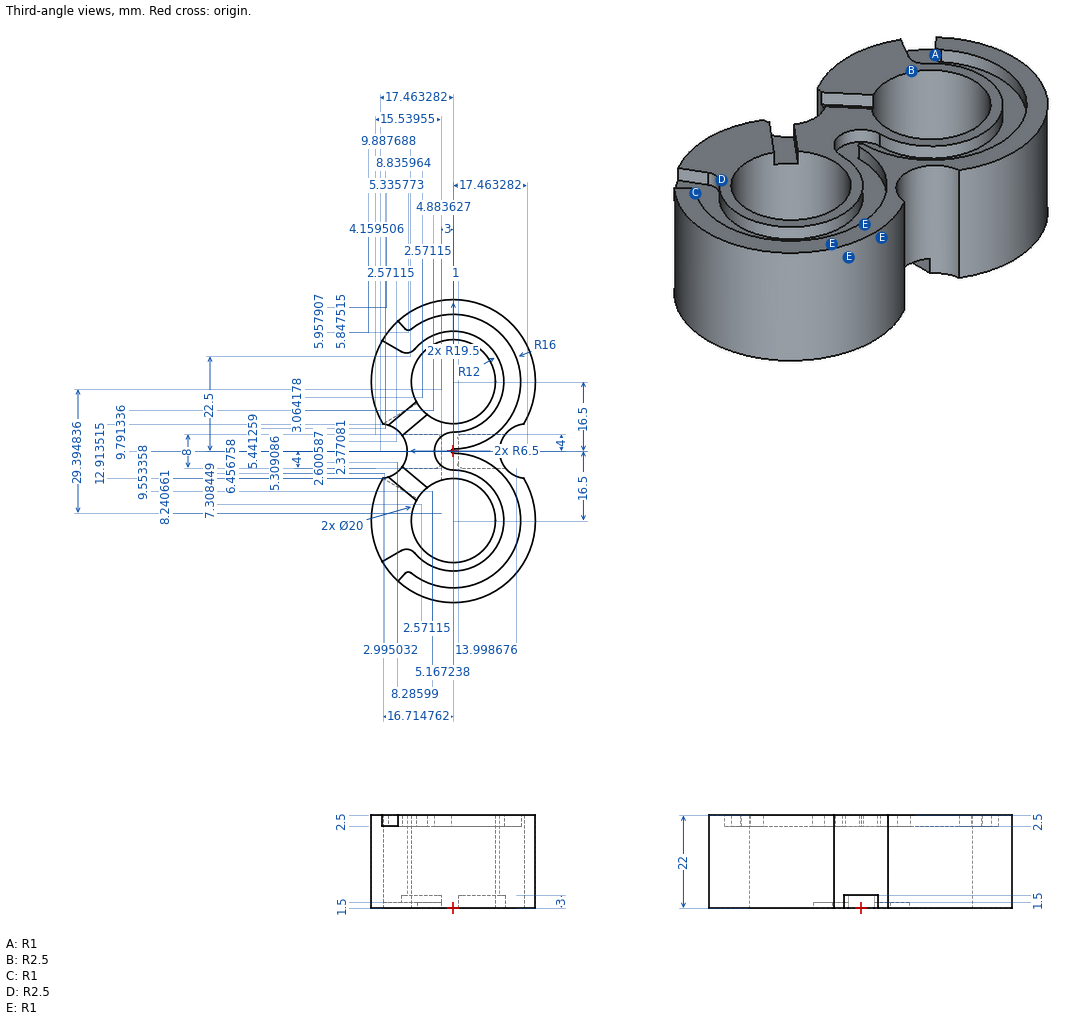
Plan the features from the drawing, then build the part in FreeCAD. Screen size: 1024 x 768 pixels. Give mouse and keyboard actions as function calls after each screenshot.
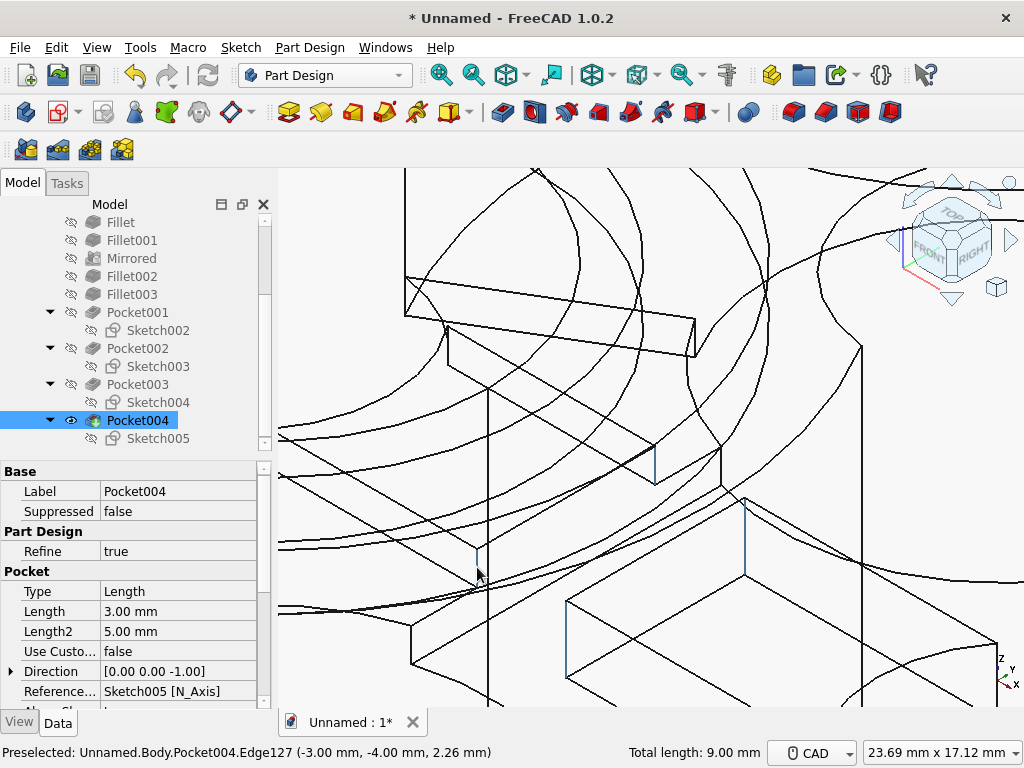
key(v)
key(1)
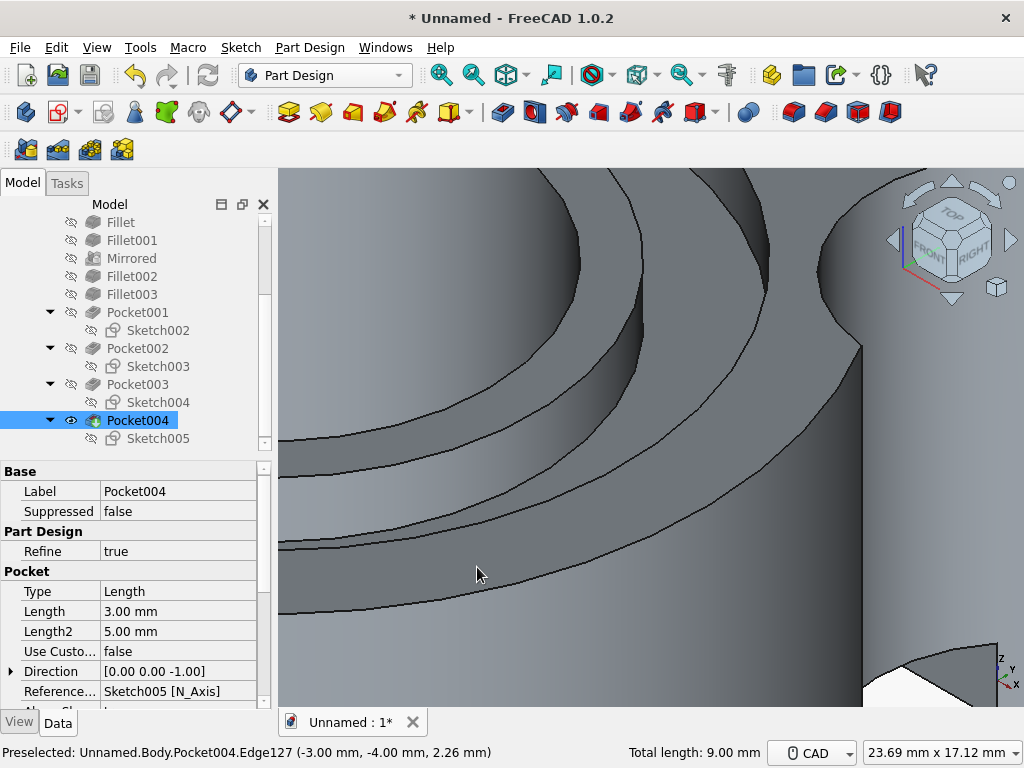
click(794, 112)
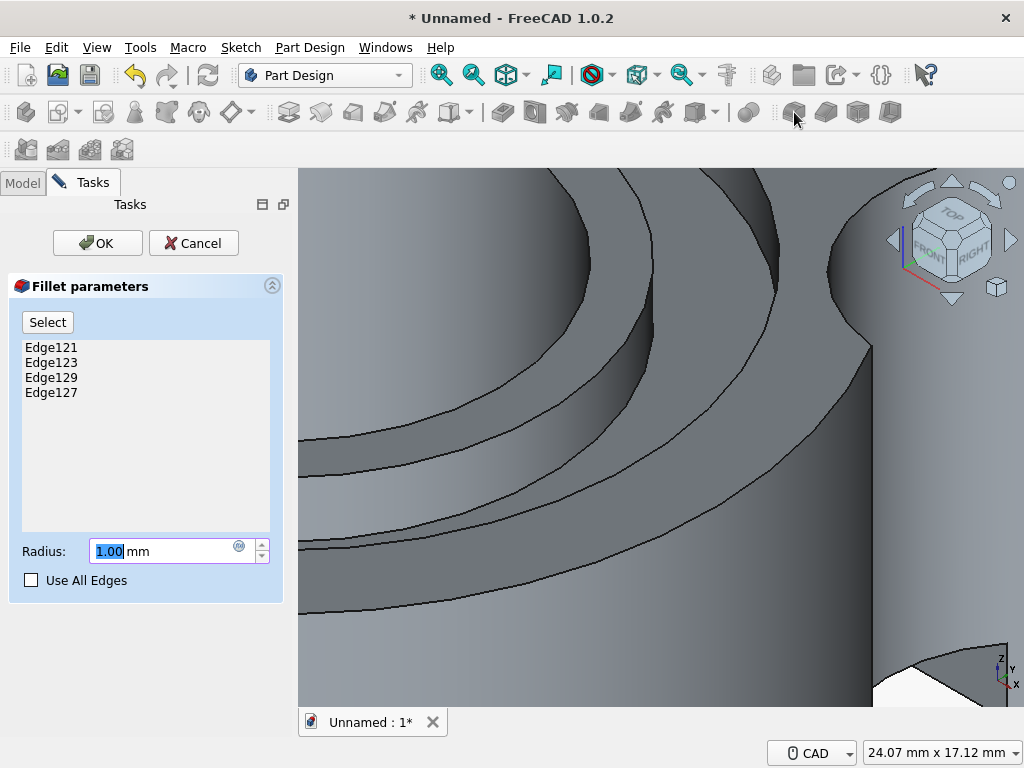
text(1)
key(Tab)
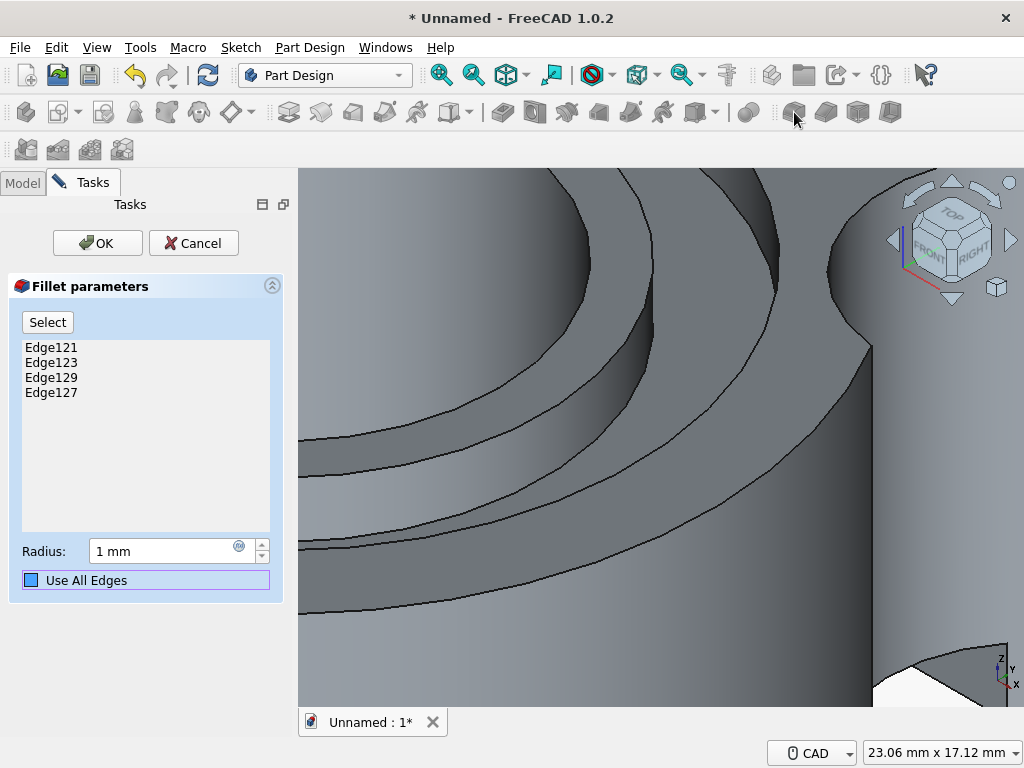
click(98, 243)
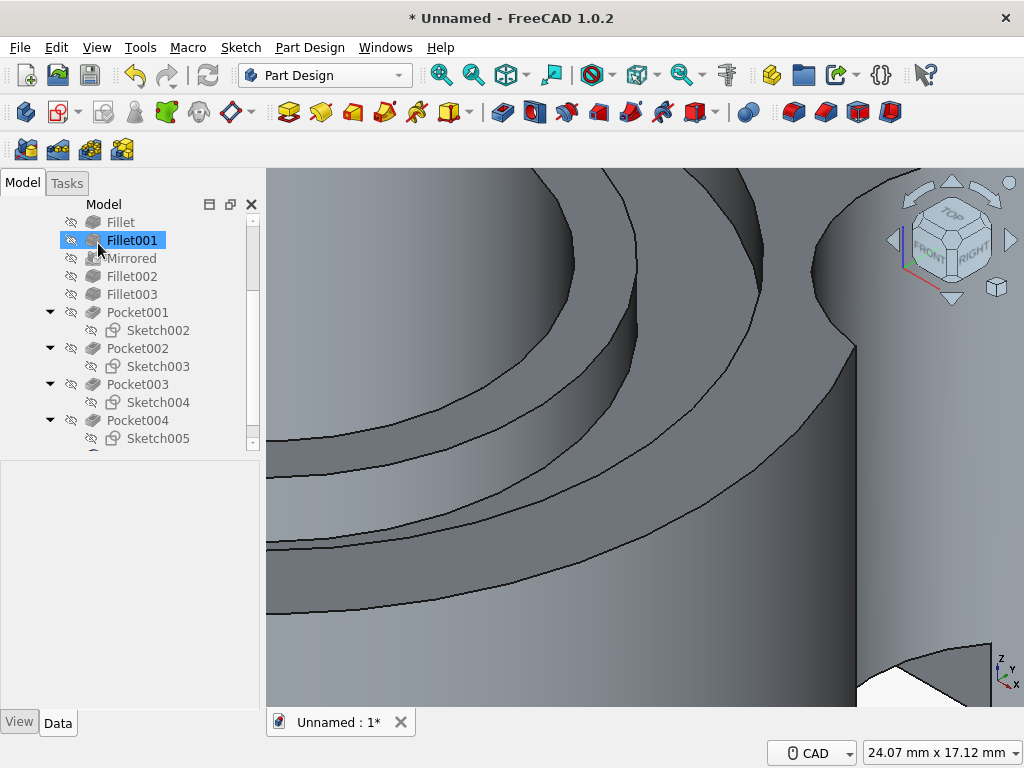
key(v)
key(f)